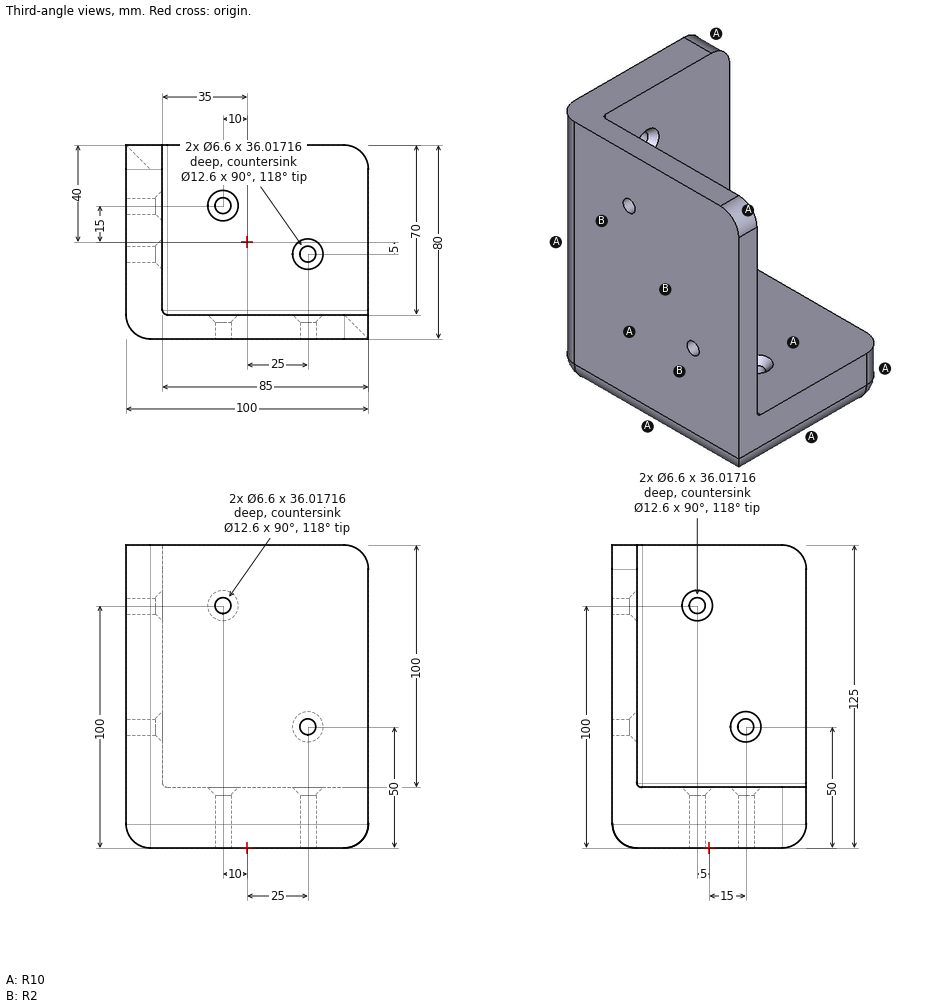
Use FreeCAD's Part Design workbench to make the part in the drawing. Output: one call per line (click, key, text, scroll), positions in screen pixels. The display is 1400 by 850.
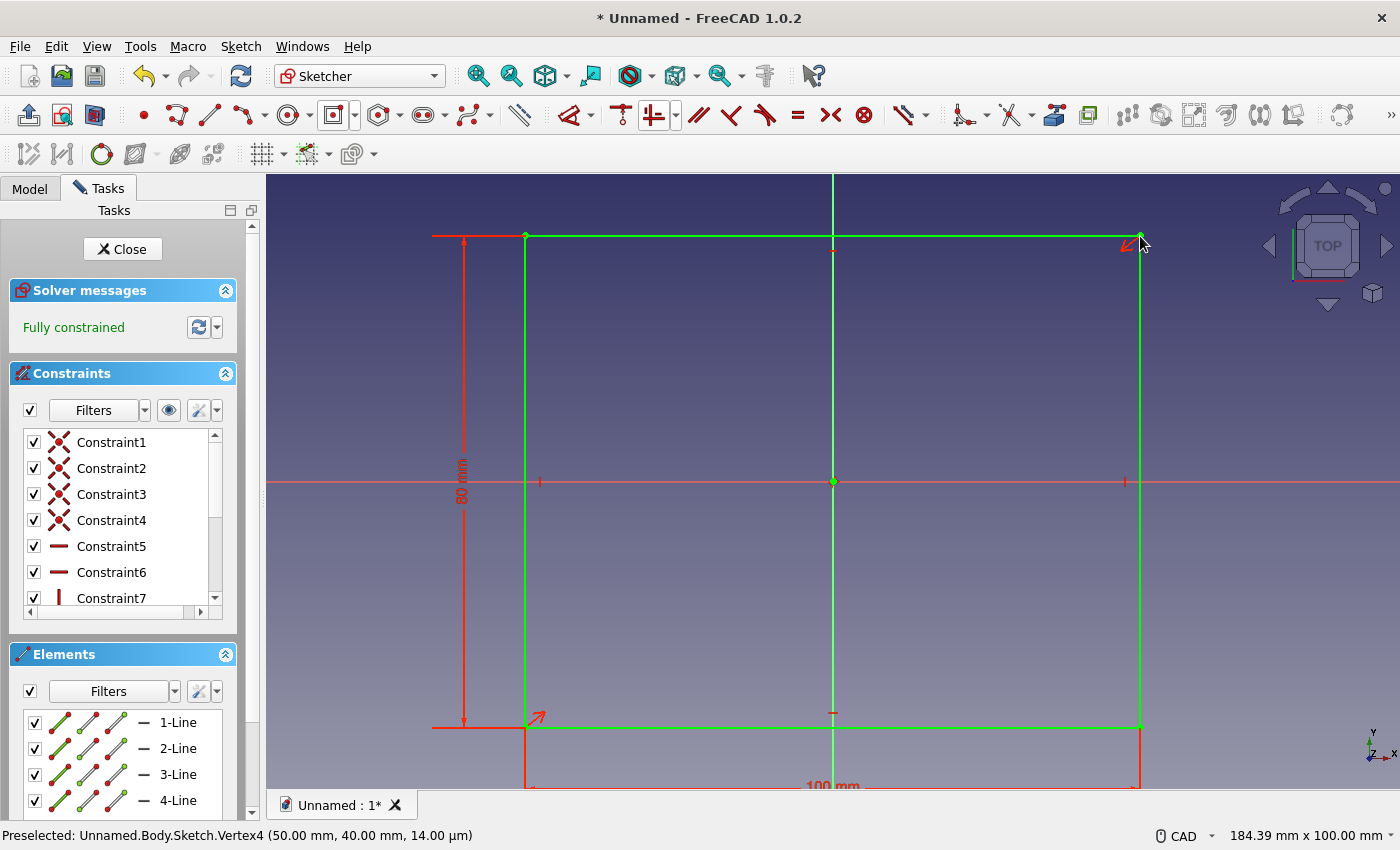
click(123, 249)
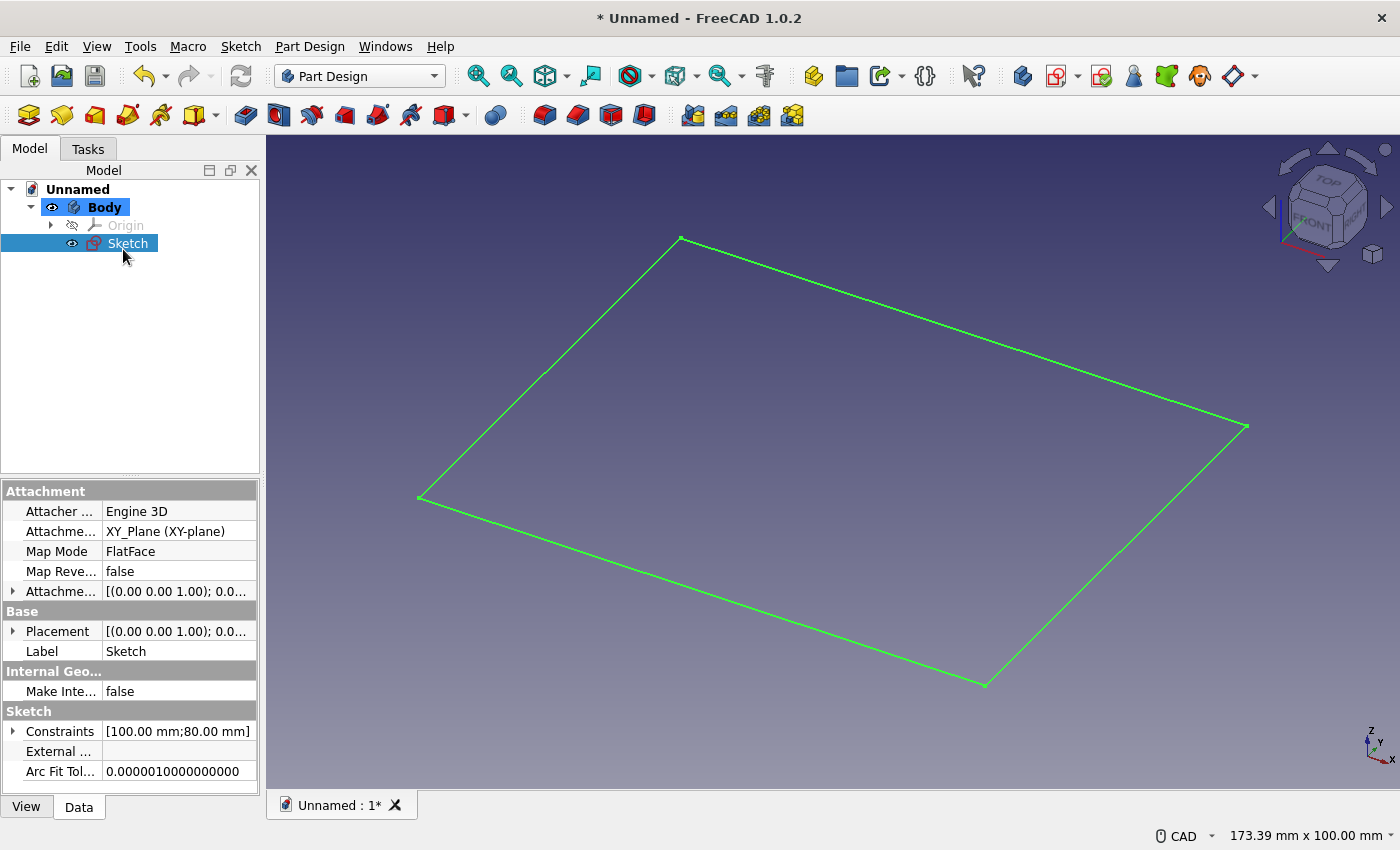
click(29, 116)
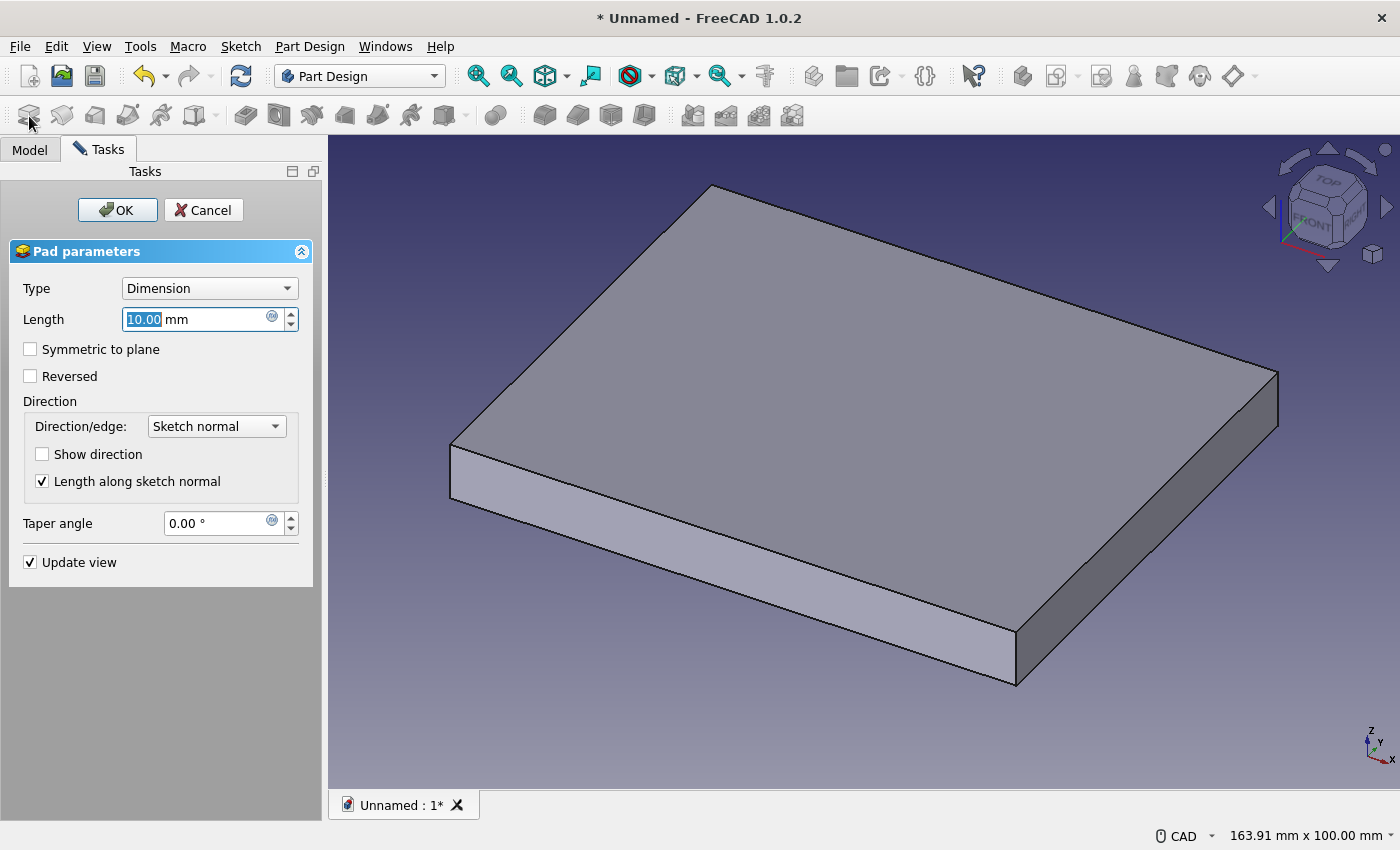
text(125)
key(Tab)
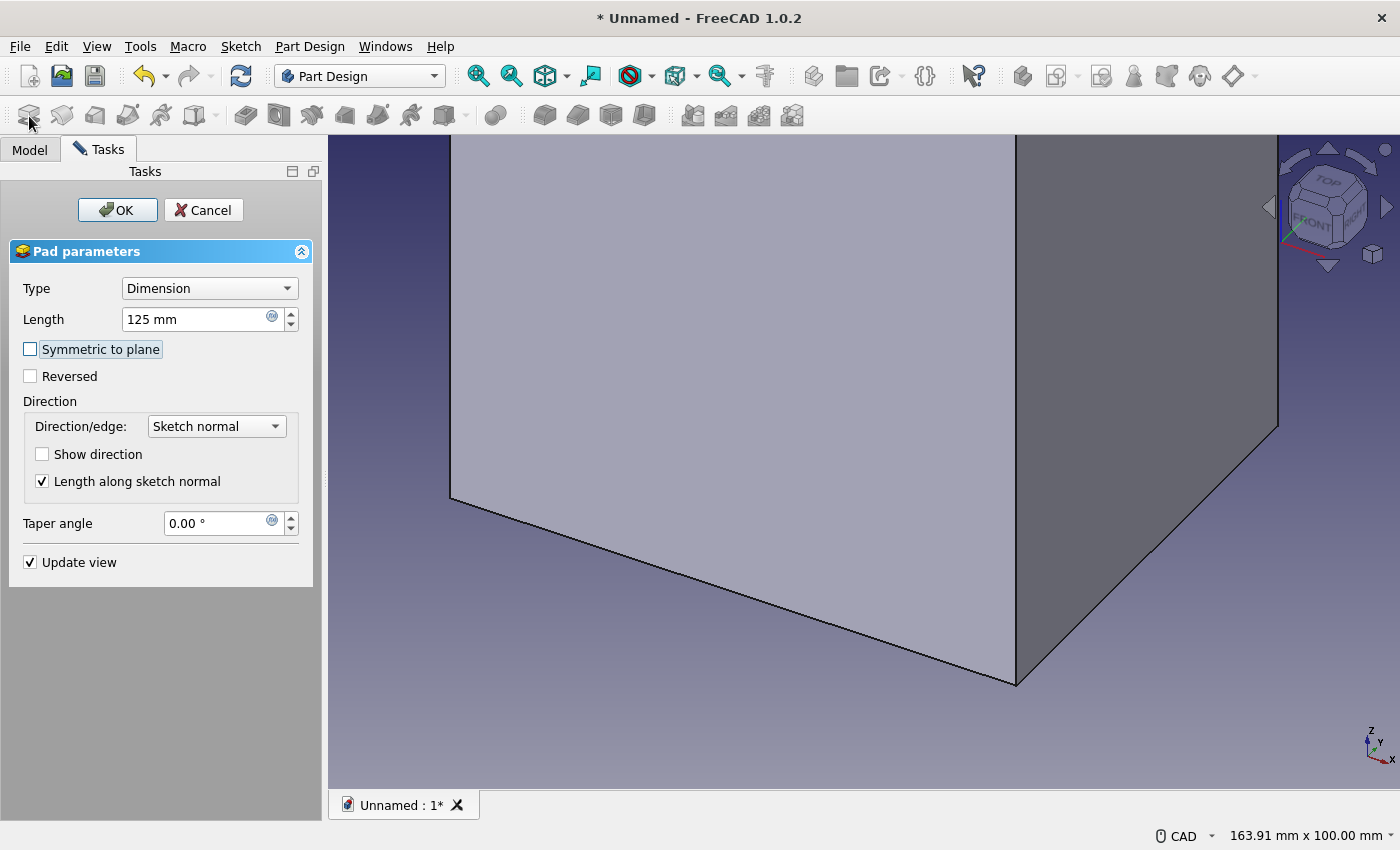
click(118, 210)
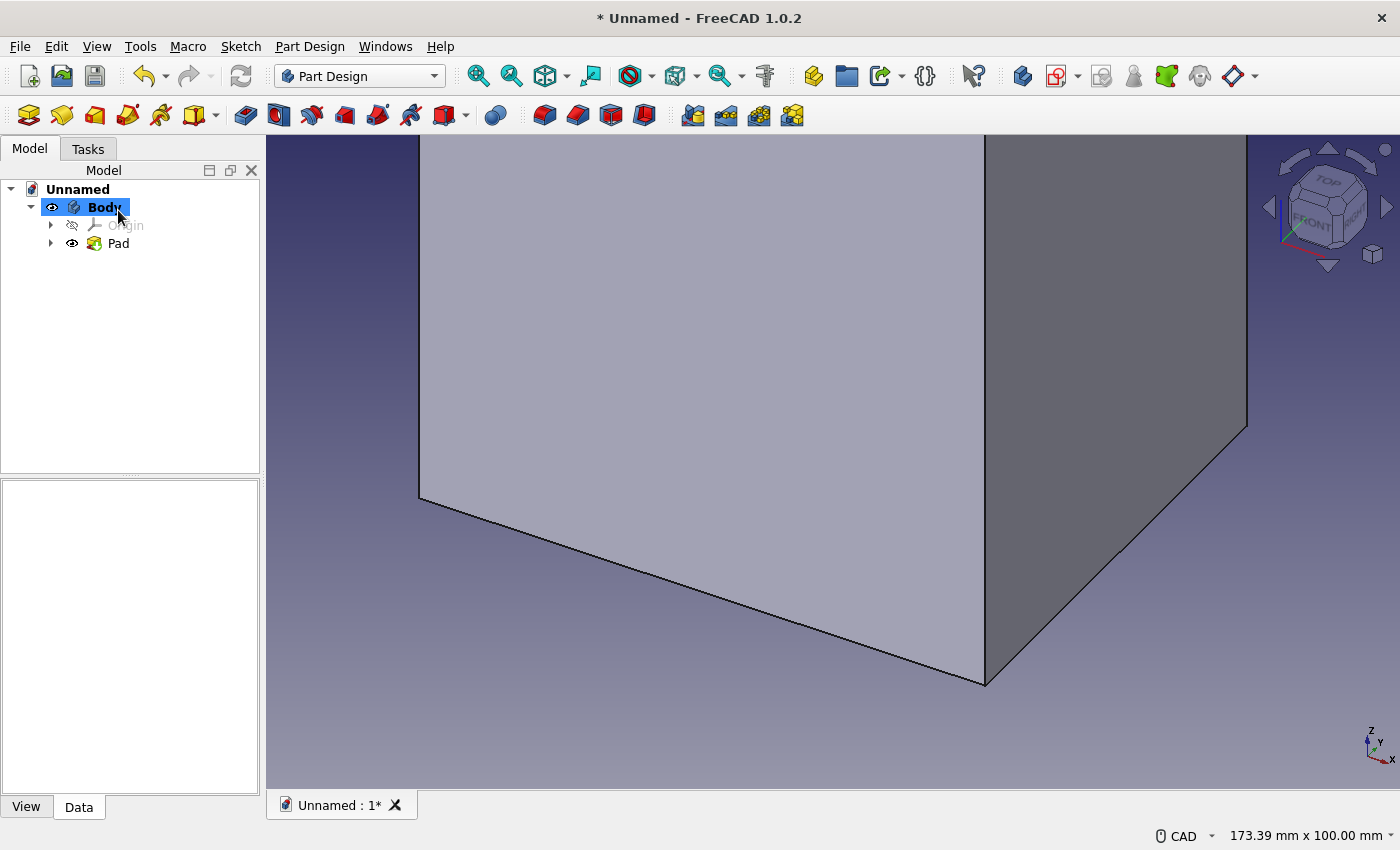
key(v)
key(f)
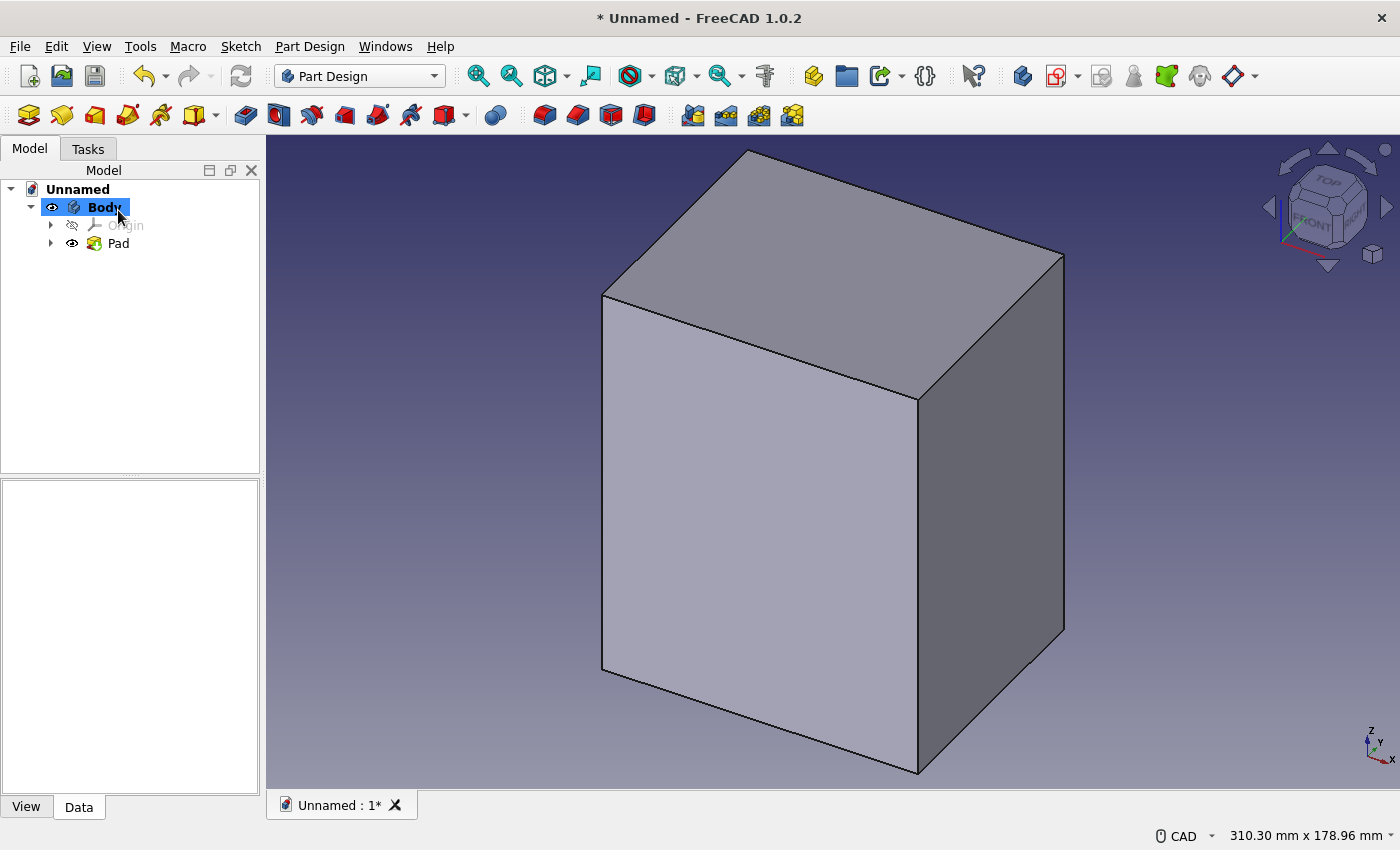
click(833, 274)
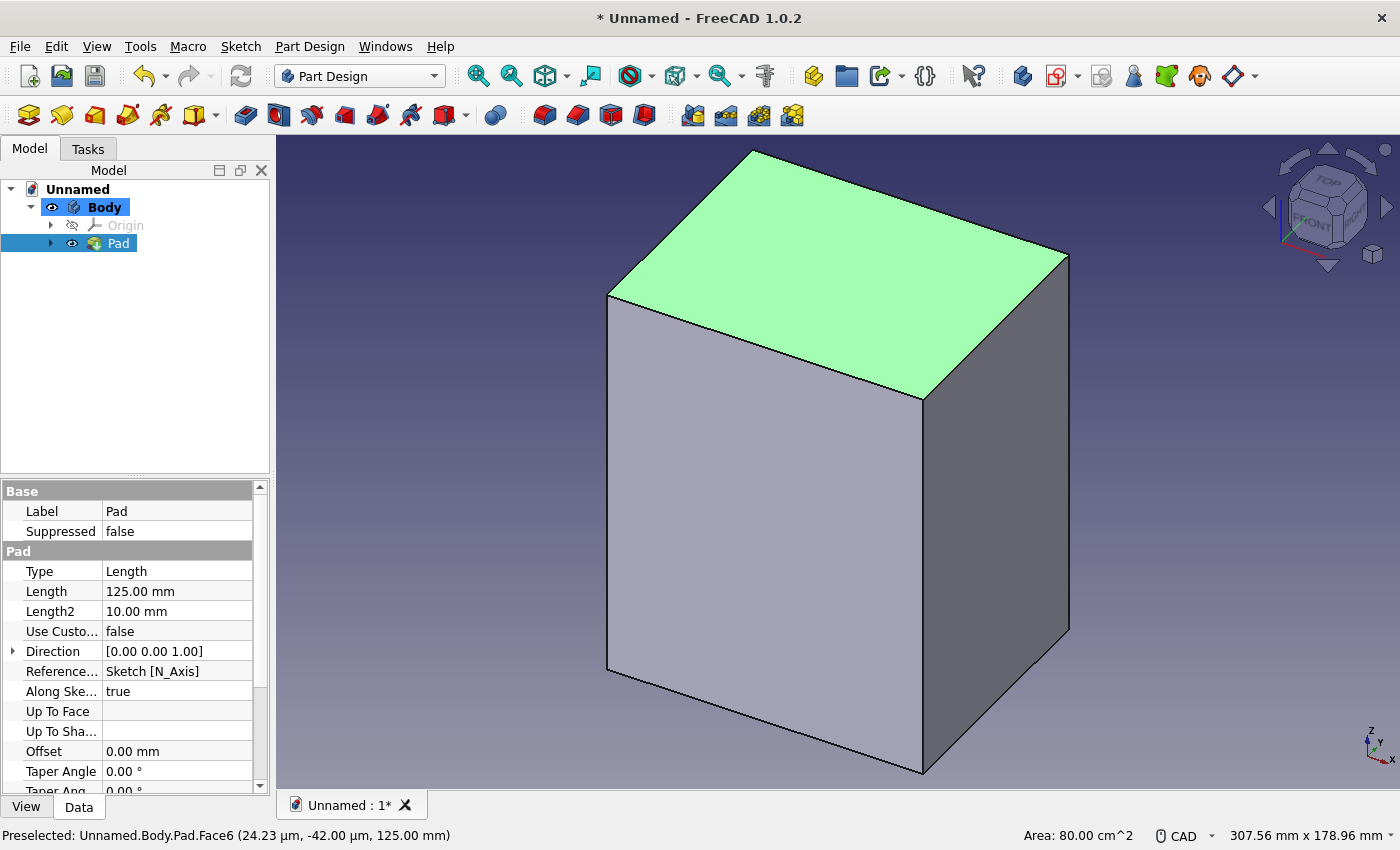
click(1056, 76)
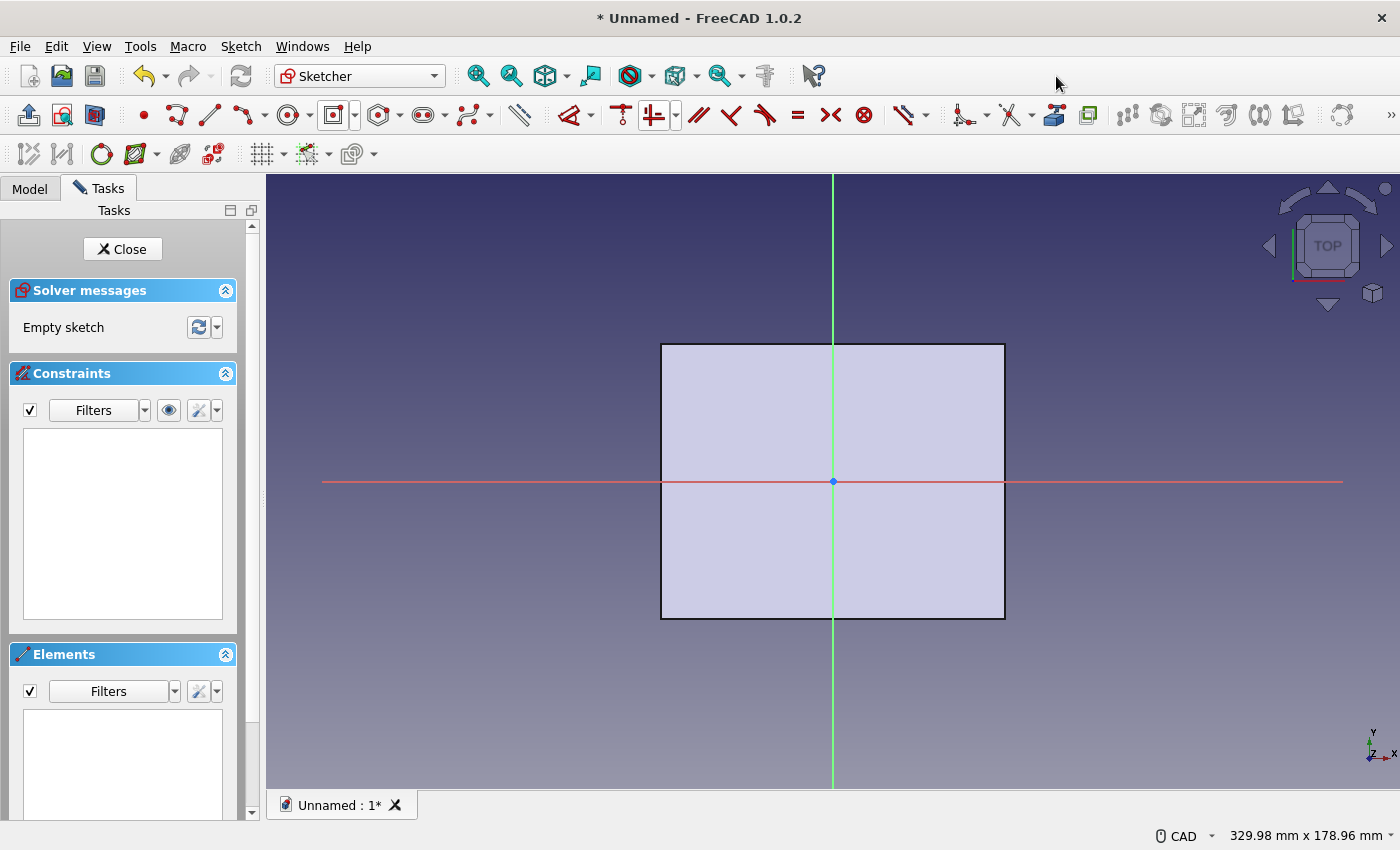
scroll(1050, 429, up, 2)